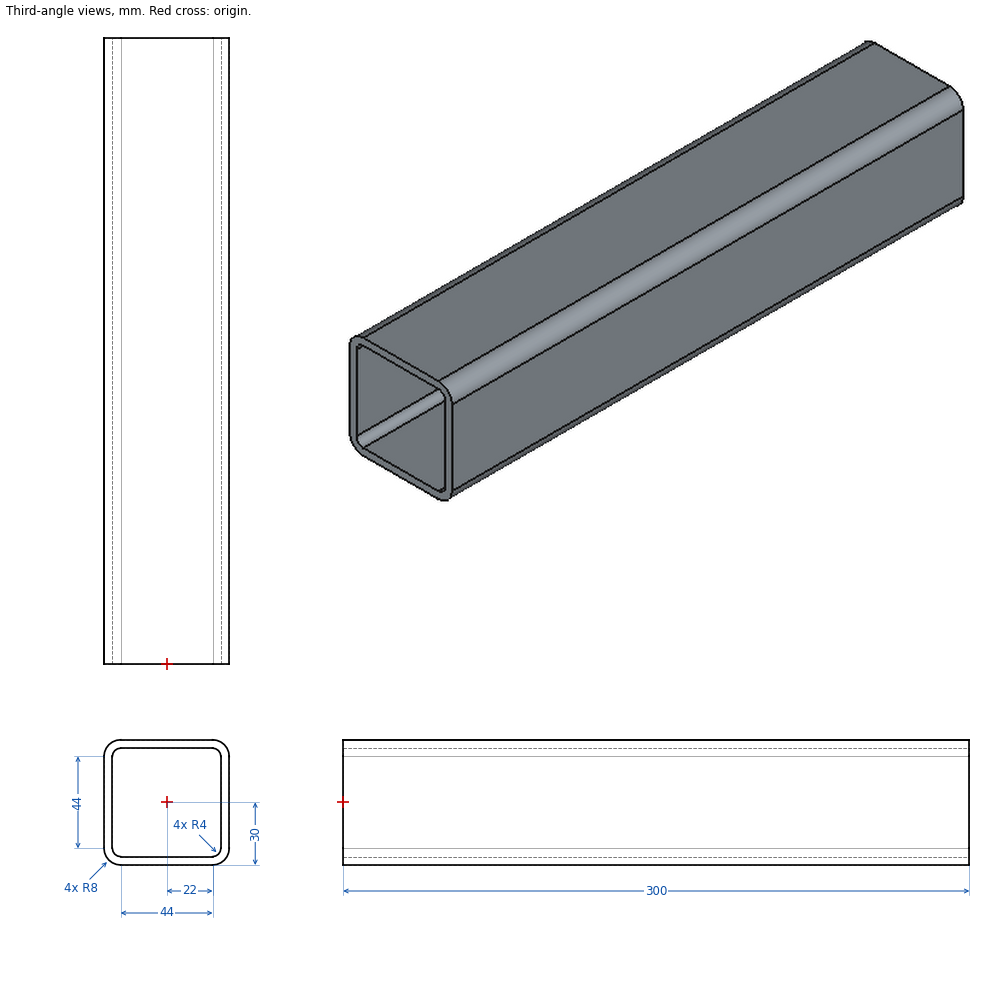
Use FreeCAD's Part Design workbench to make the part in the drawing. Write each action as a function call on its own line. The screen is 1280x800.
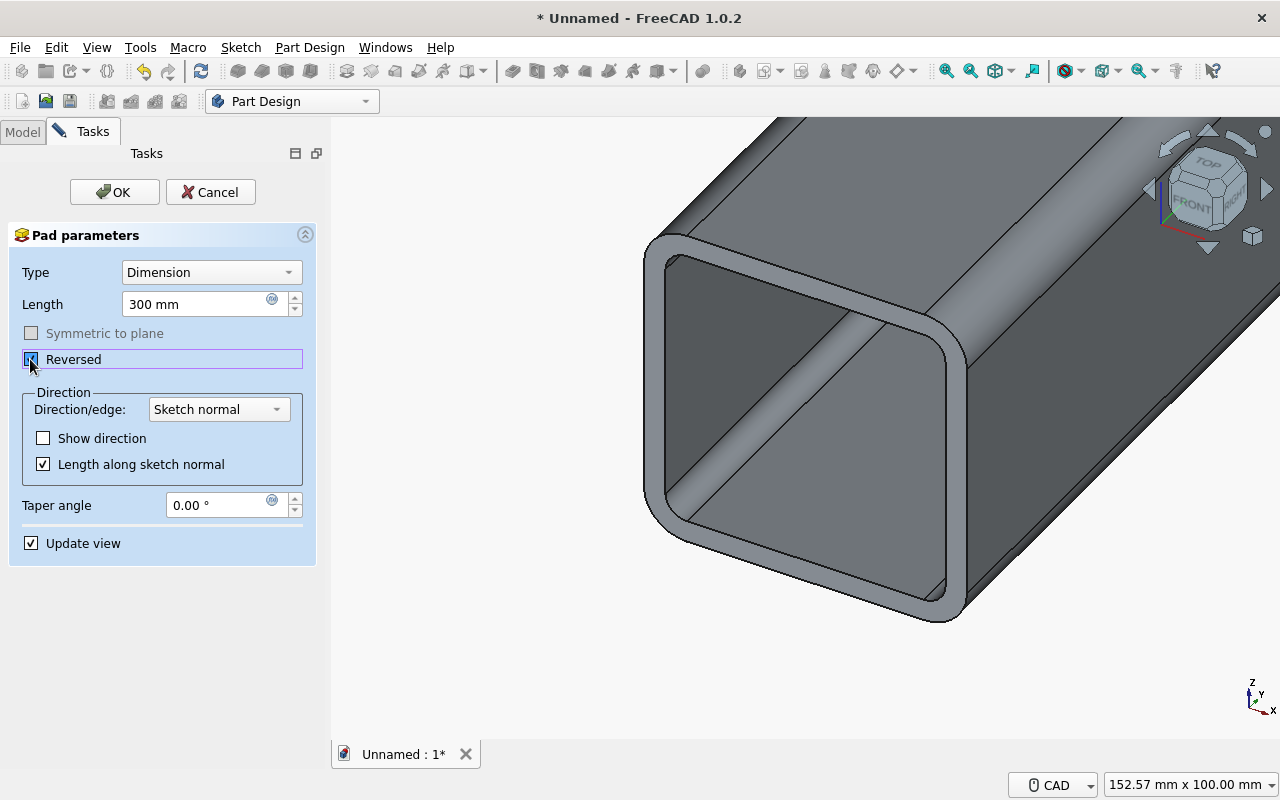
click(115, 192)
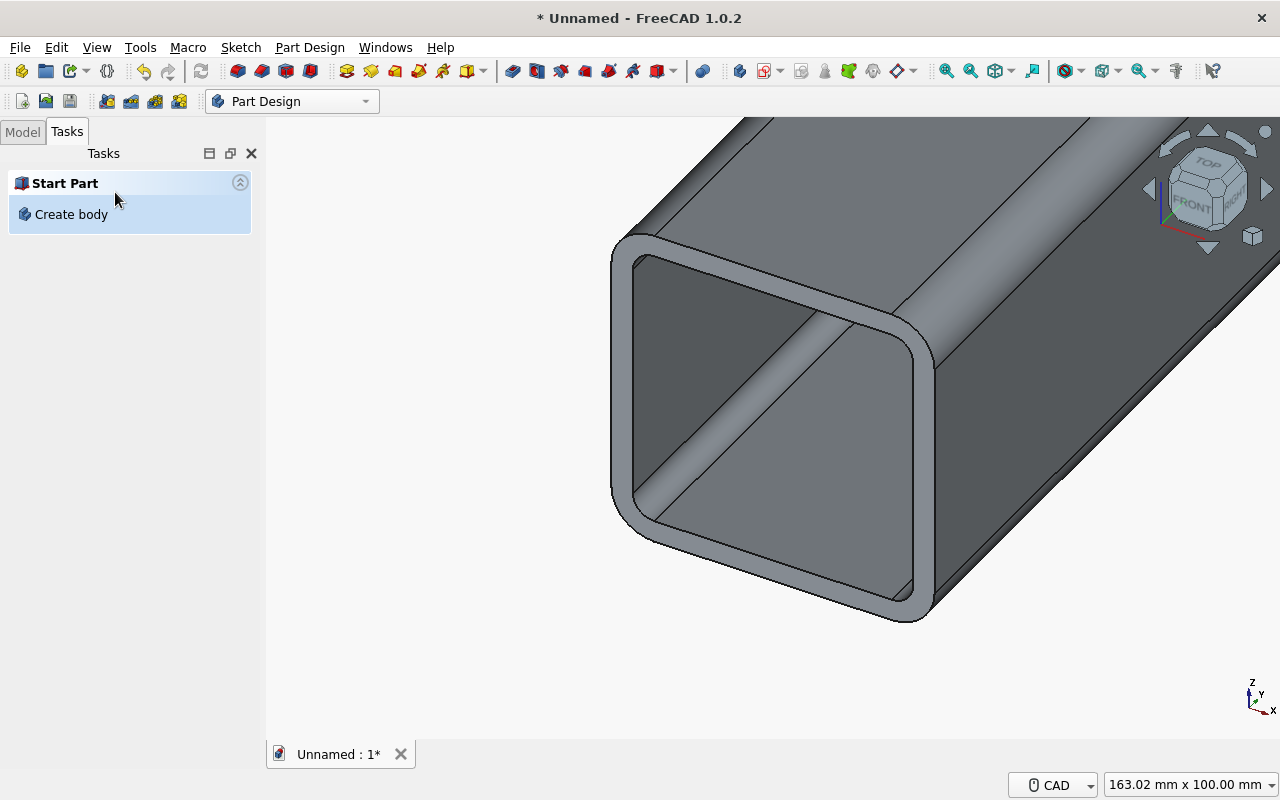
key(0)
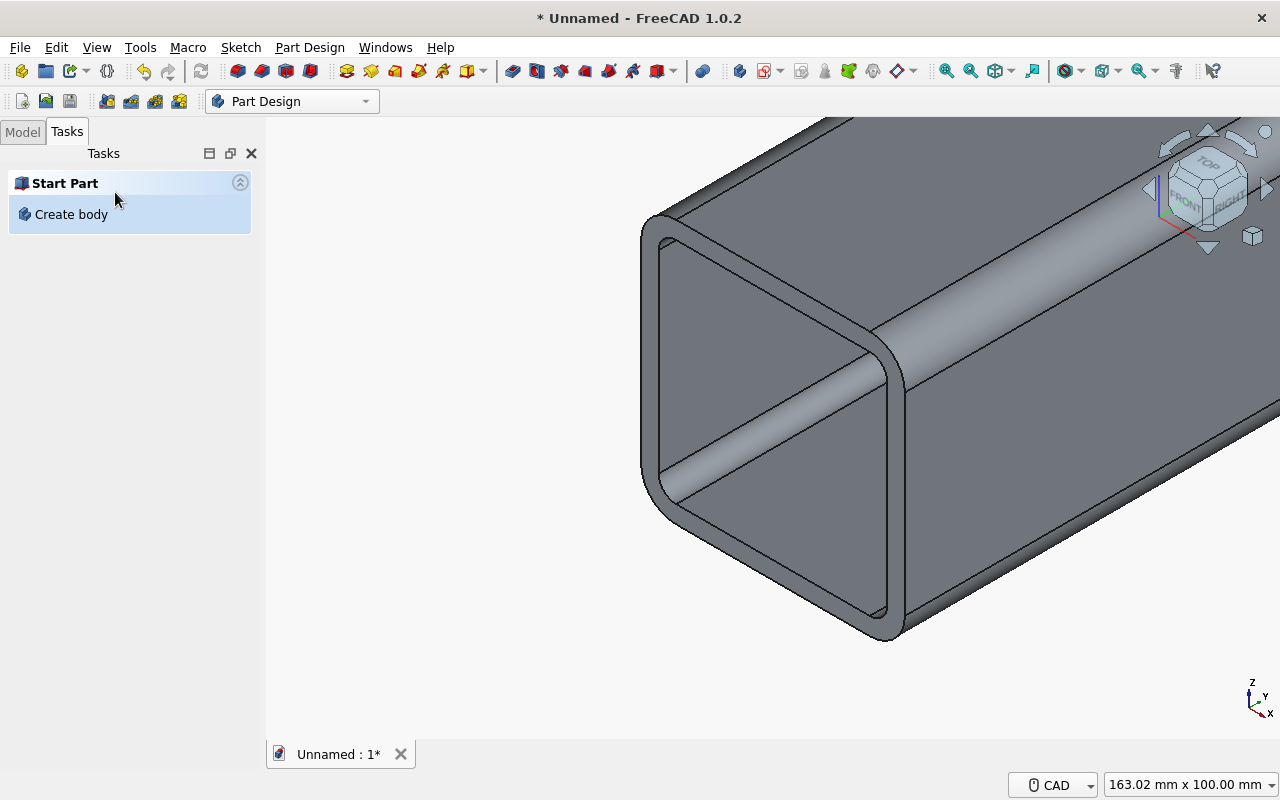
key(v)
key(f)